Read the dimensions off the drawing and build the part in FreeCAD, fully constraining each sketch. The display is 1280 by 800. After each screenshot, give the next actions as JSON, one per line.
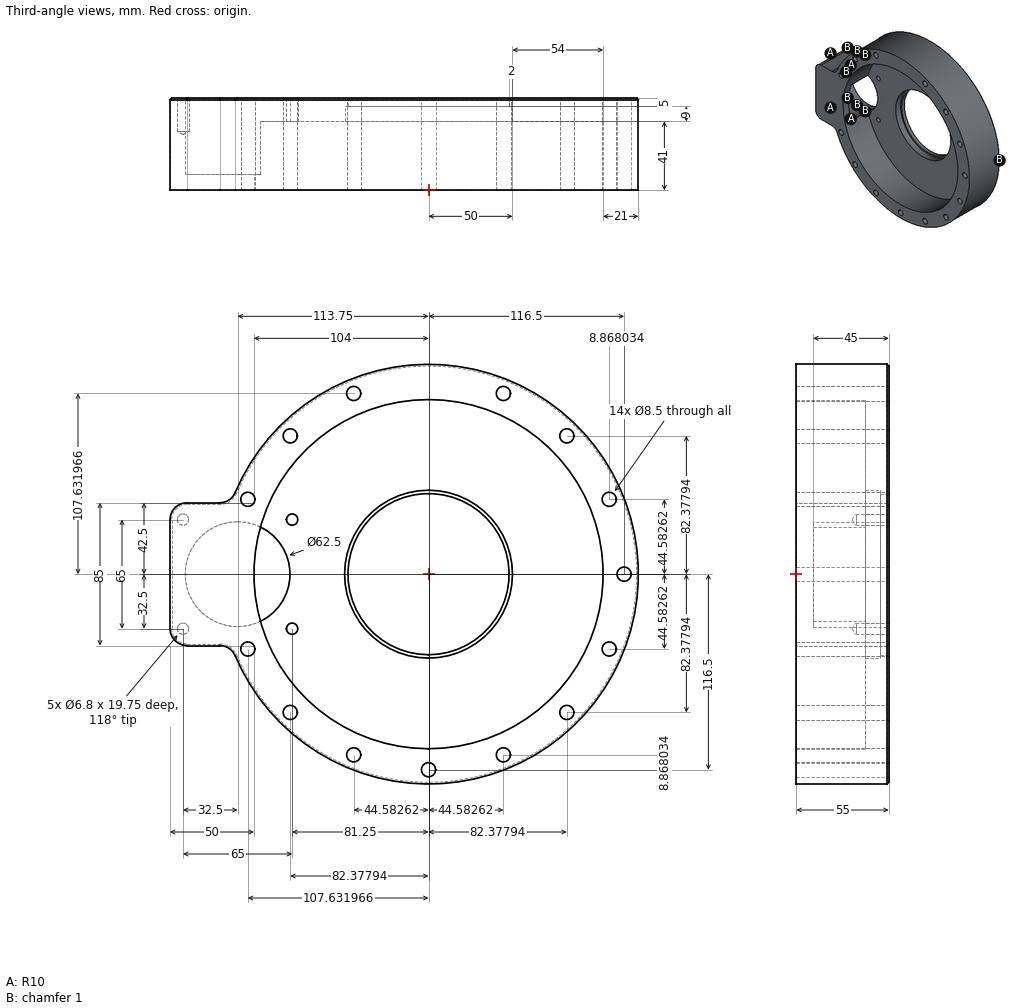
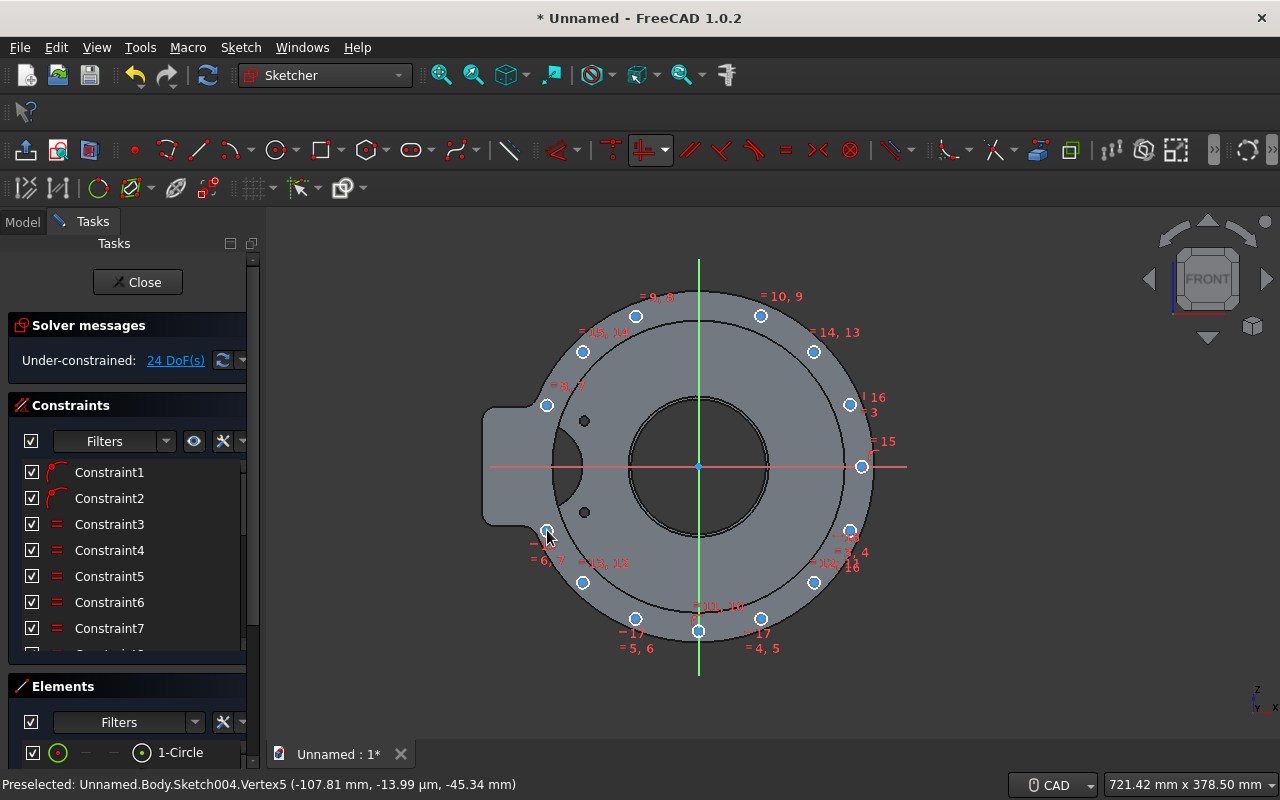
{"action": "left_click", "coordinate": [547, 531]}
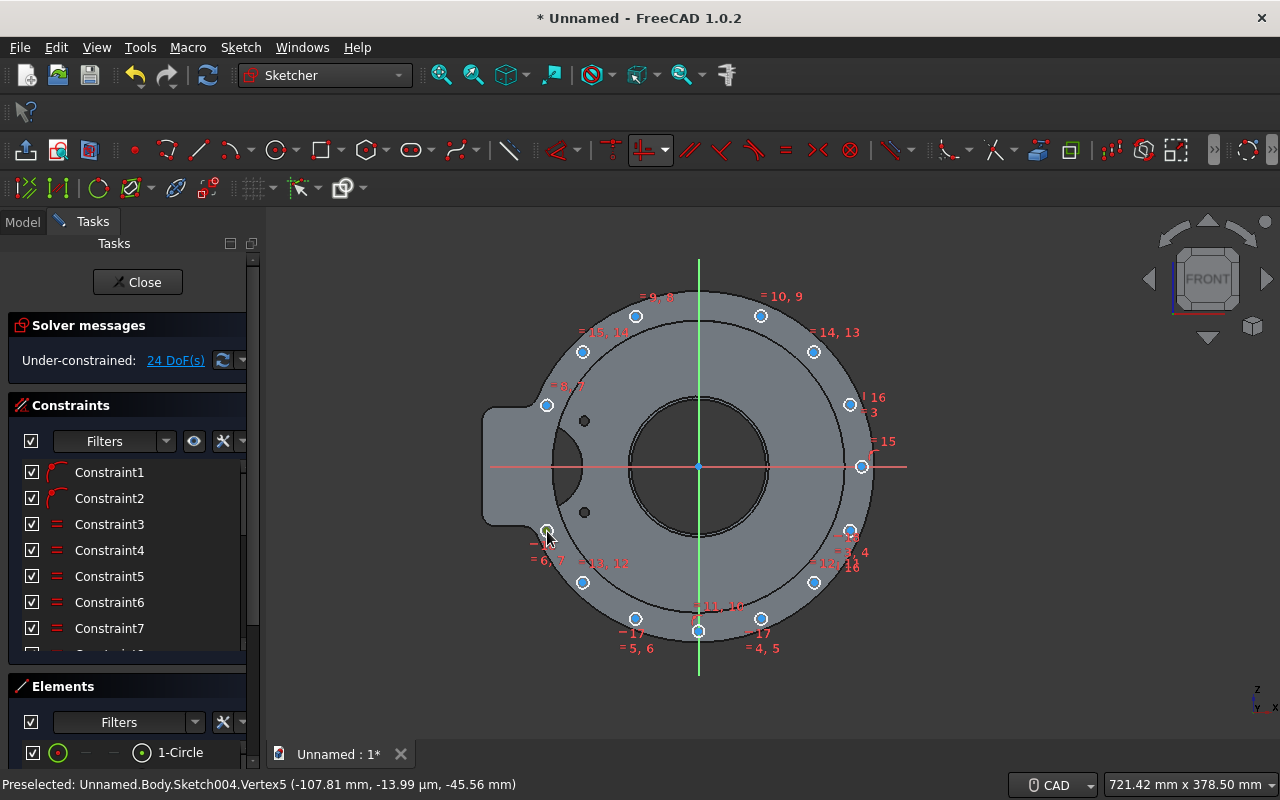
{"action": "left_click", "coordinate": [547, 405]}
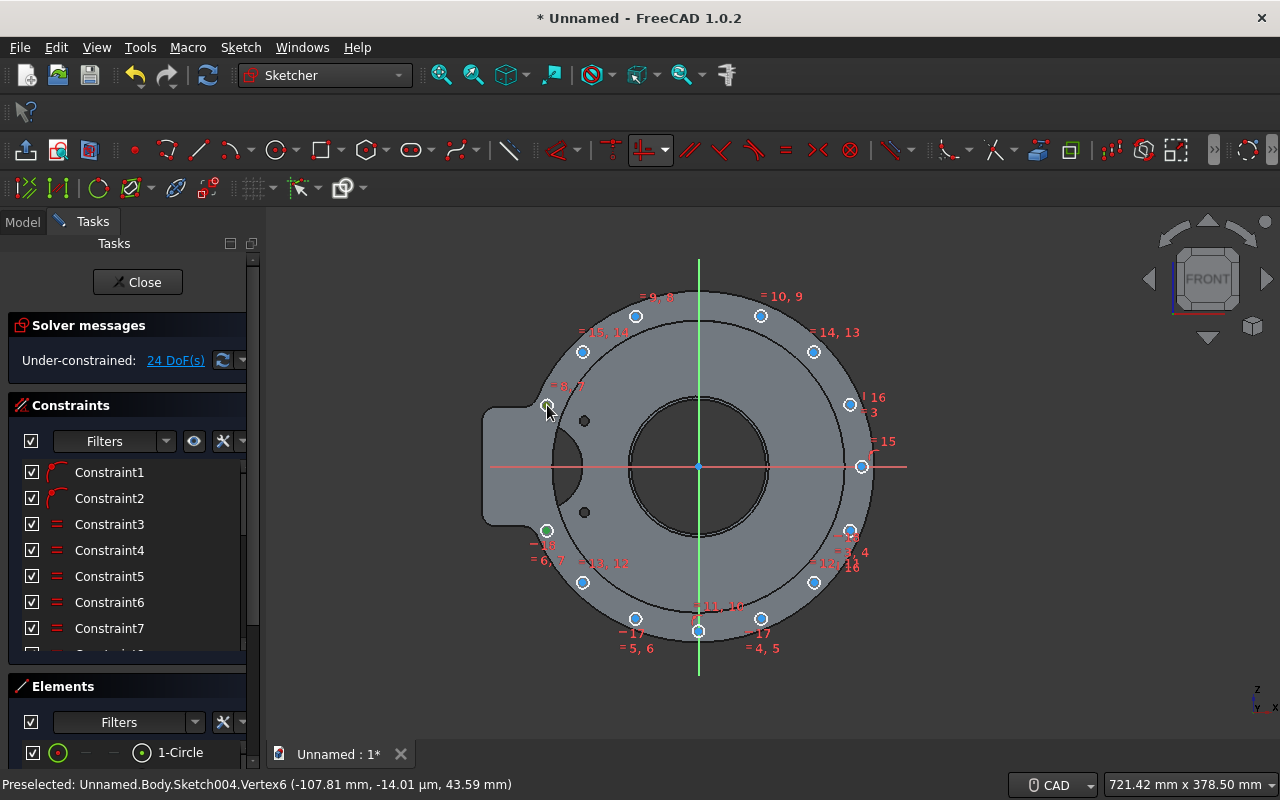
{"action": "key", "text": "v"}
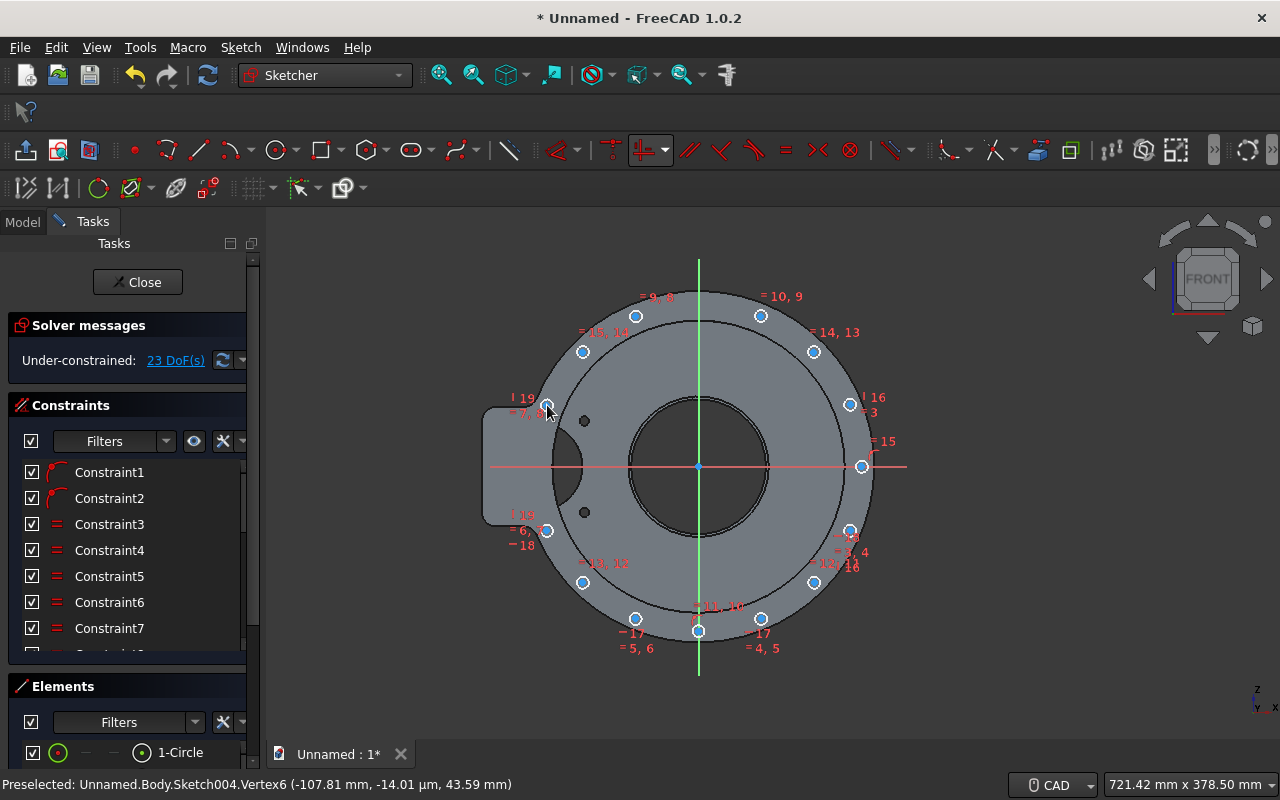
{"action": "left_click", "coordinate": [850, 405]}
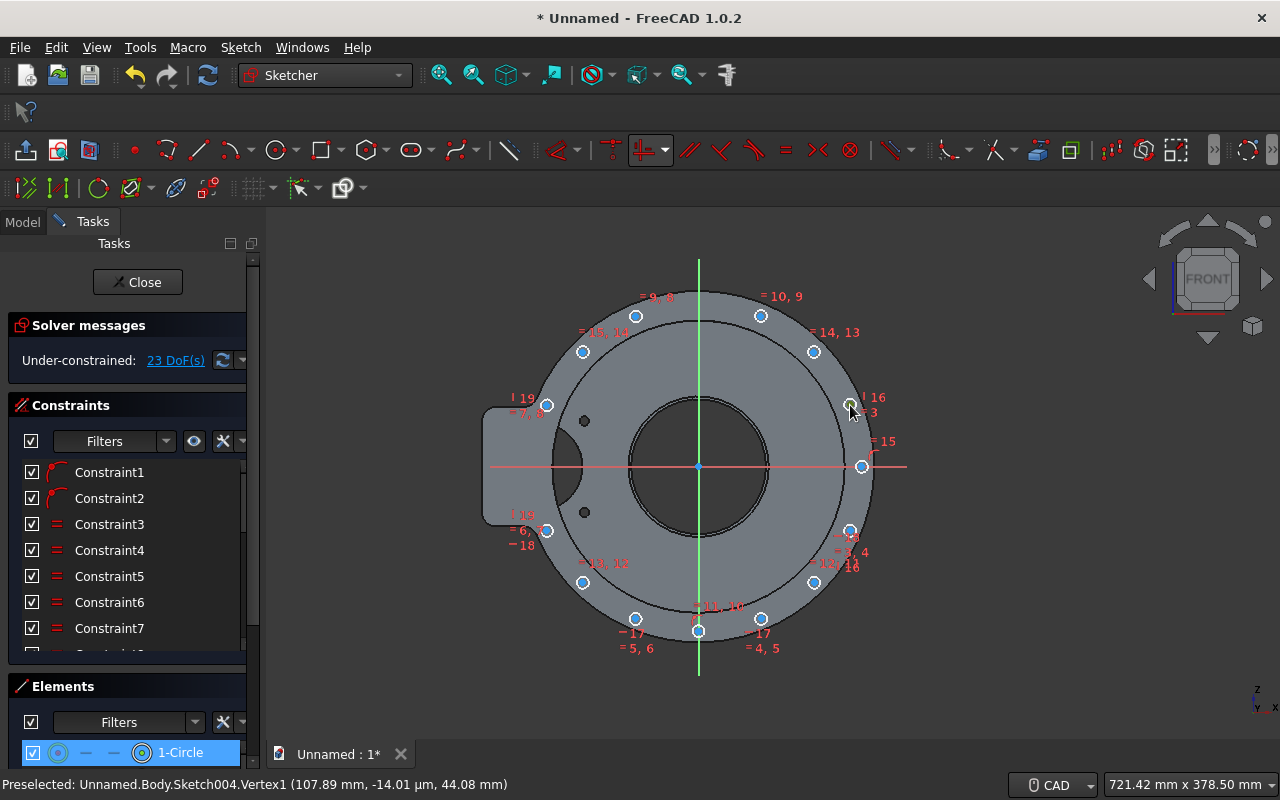
{"action": "left_click", "coordinate": [547, 405]}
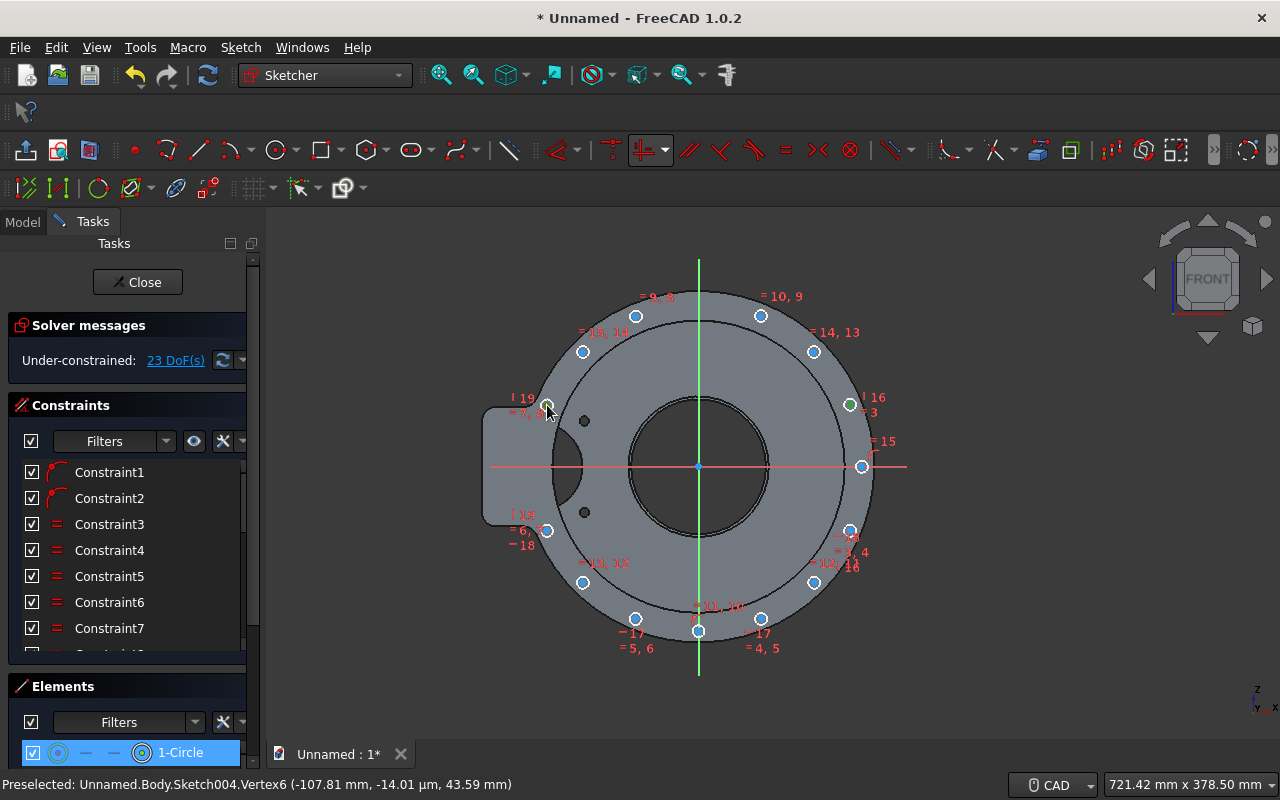
{"action": "key", "text": "h"}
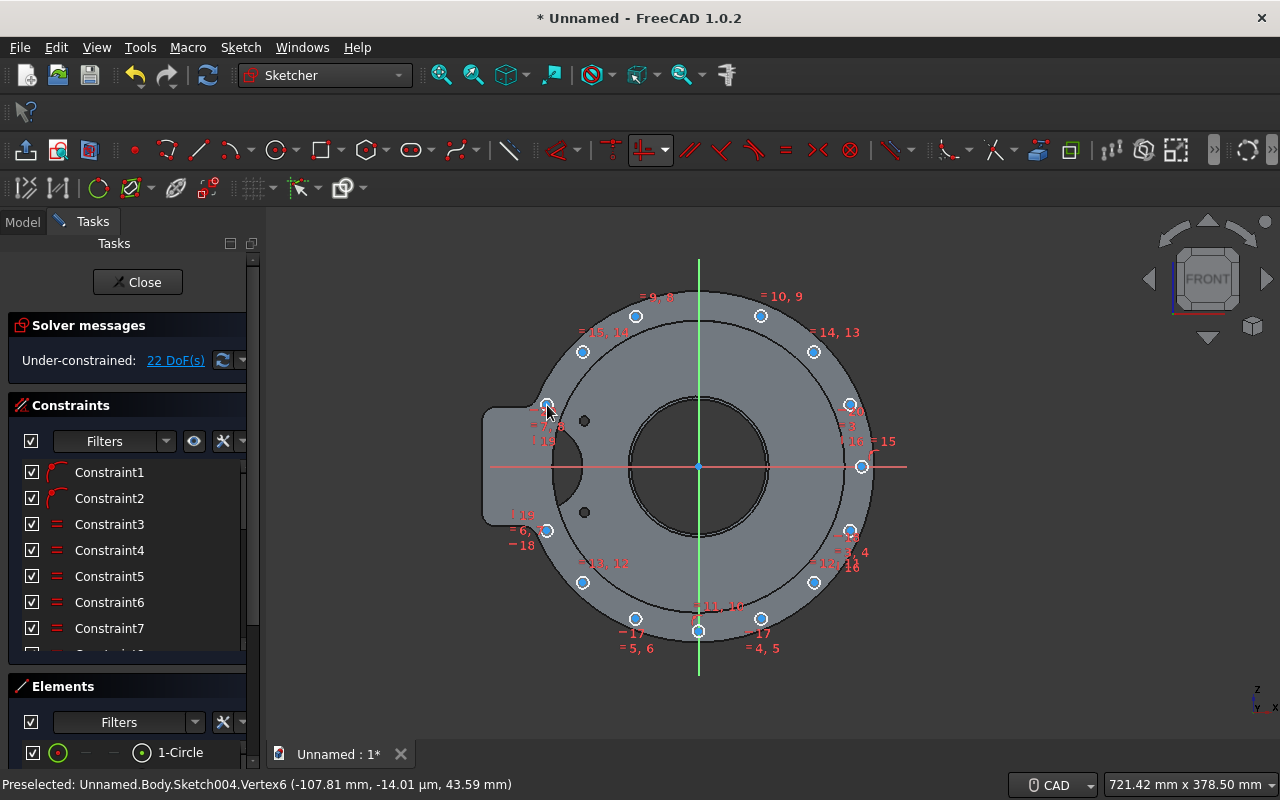
{"action": "left_click", "coordinate": [636, 619]}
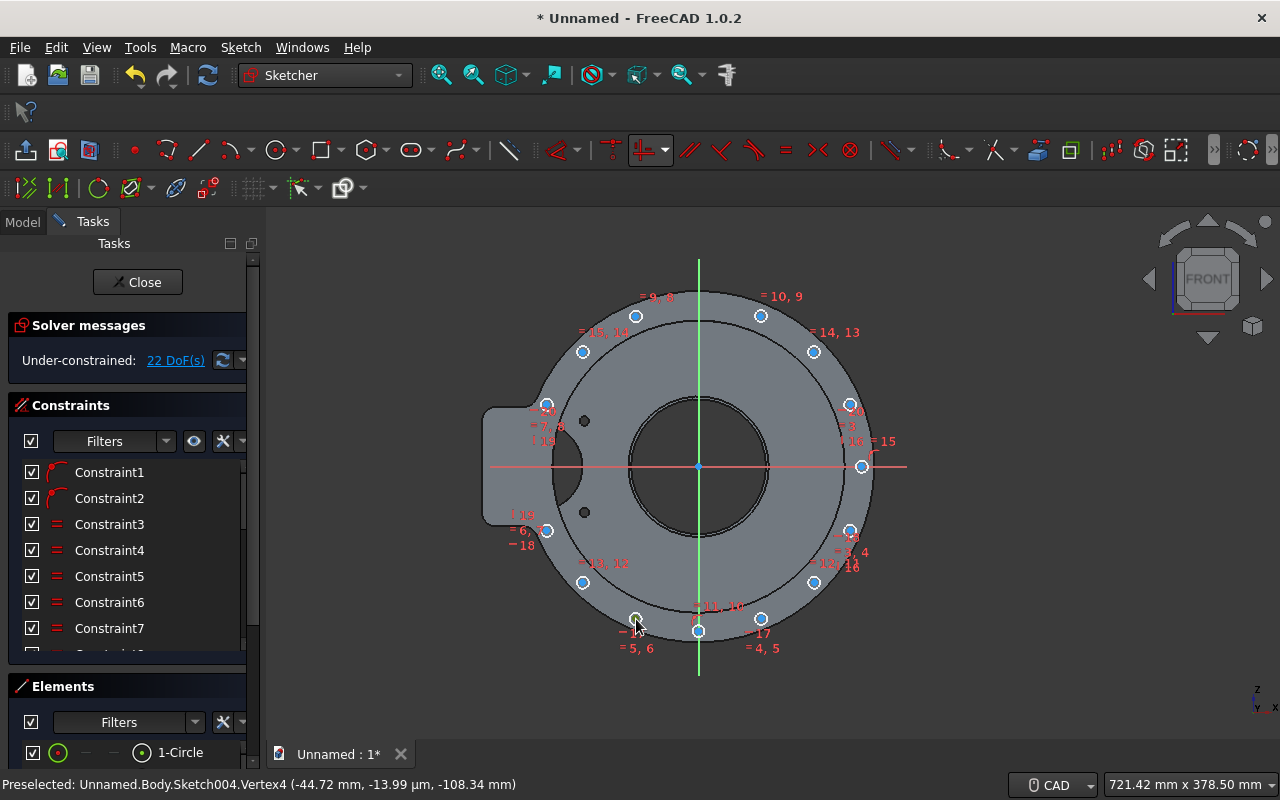
{"action": "left_click", "coordinate": [636, 316]}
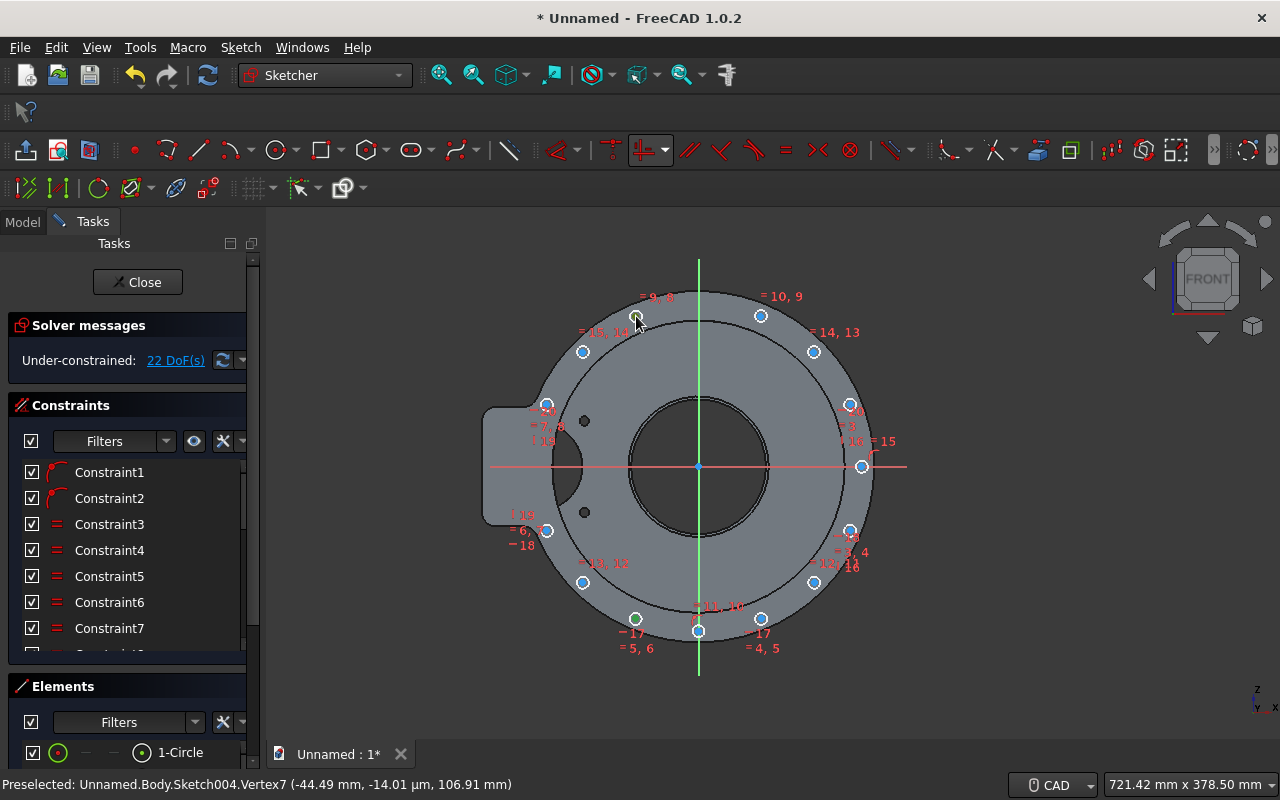
{"action": "key", "text": "v"}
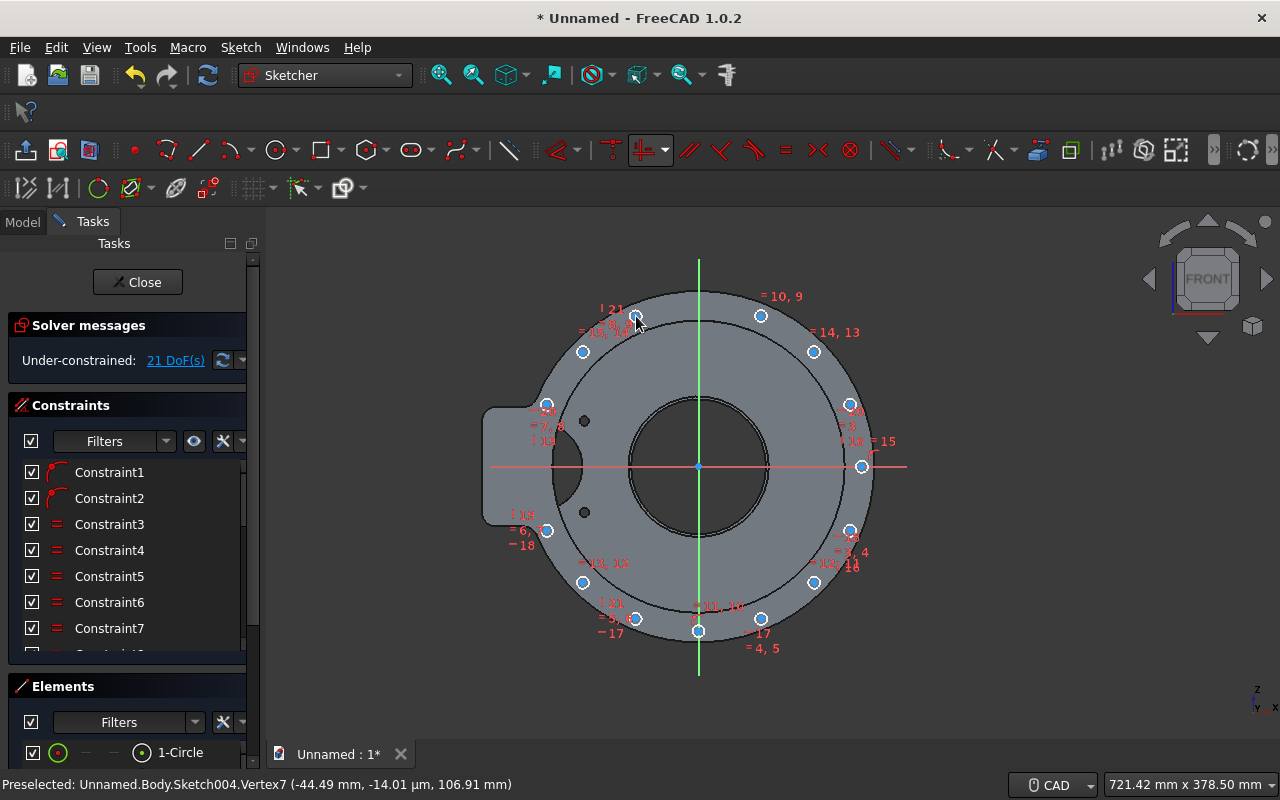
{"action": "left_click", "coordinate": [761, 619]}